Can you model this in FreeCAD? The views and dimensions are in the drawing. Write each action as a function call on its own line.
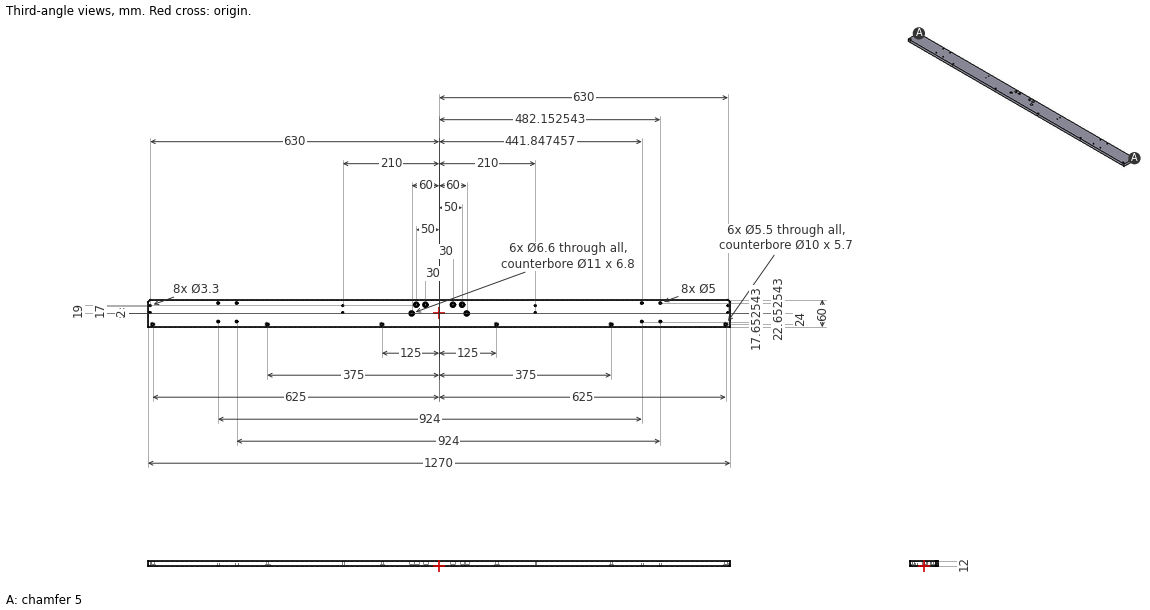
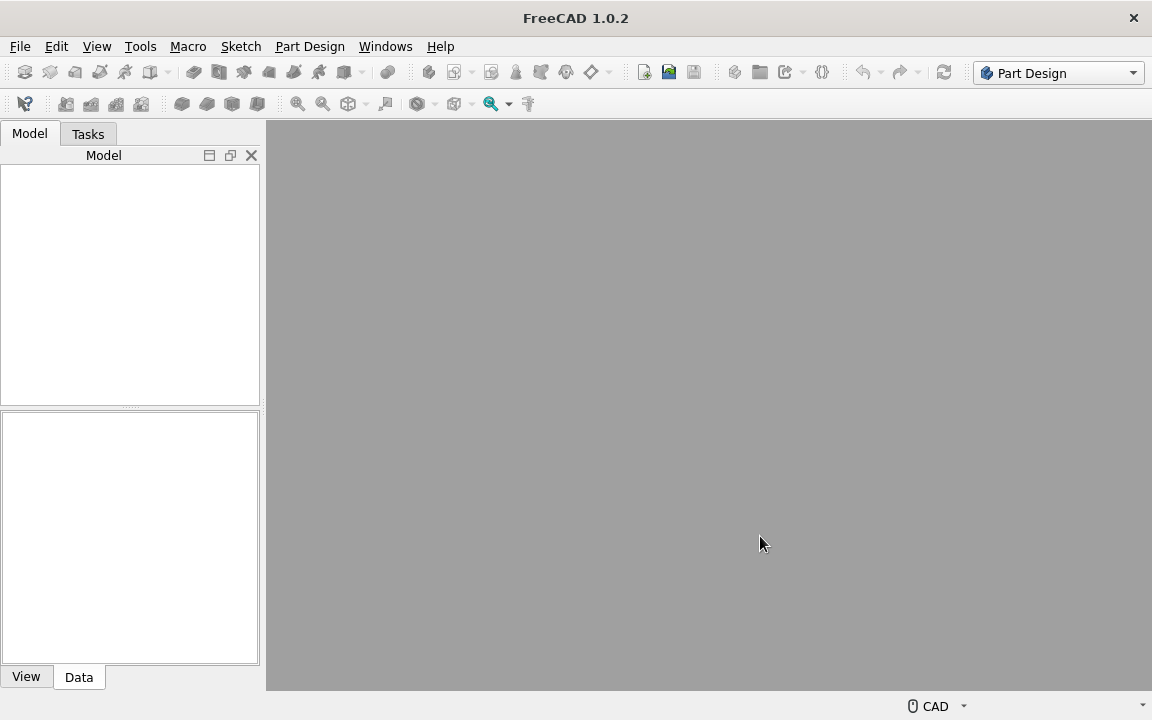
click(644, 72)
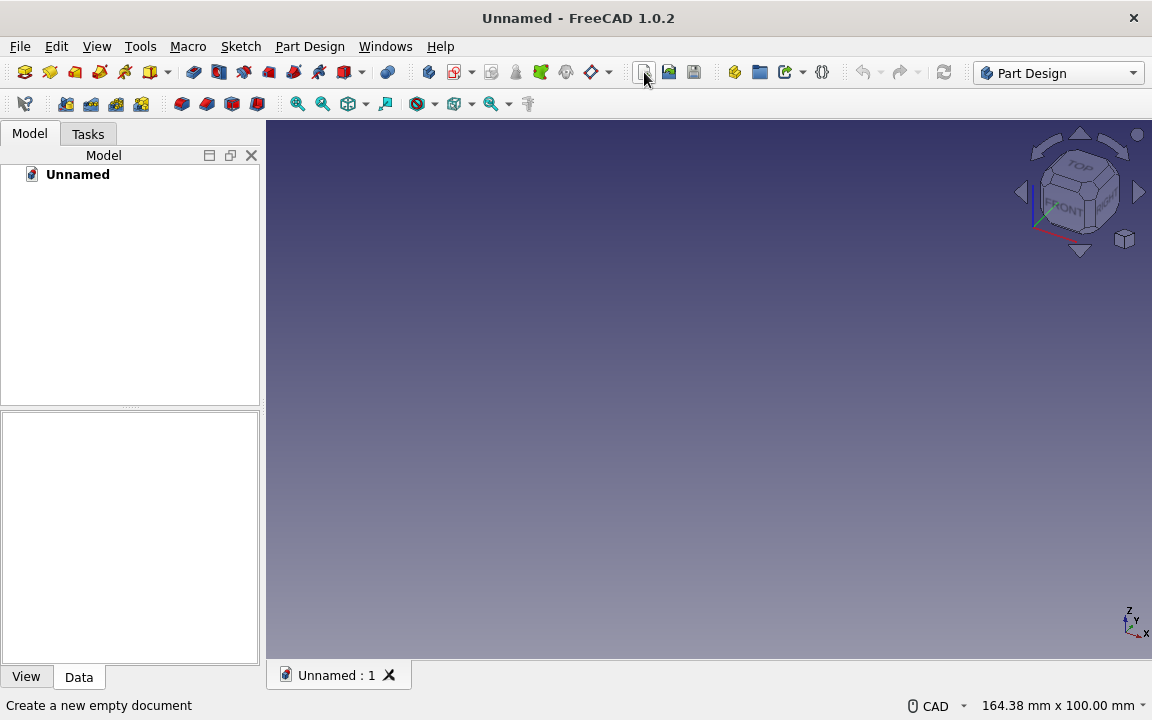
click(454, 72)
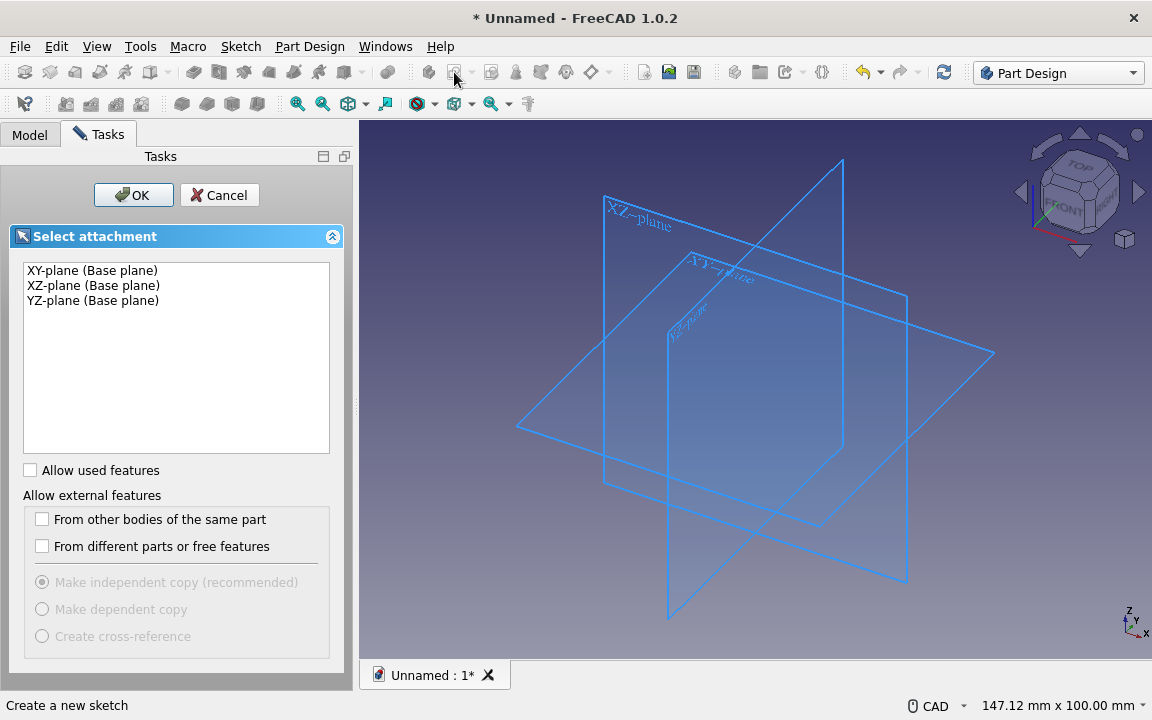
click(84, 270)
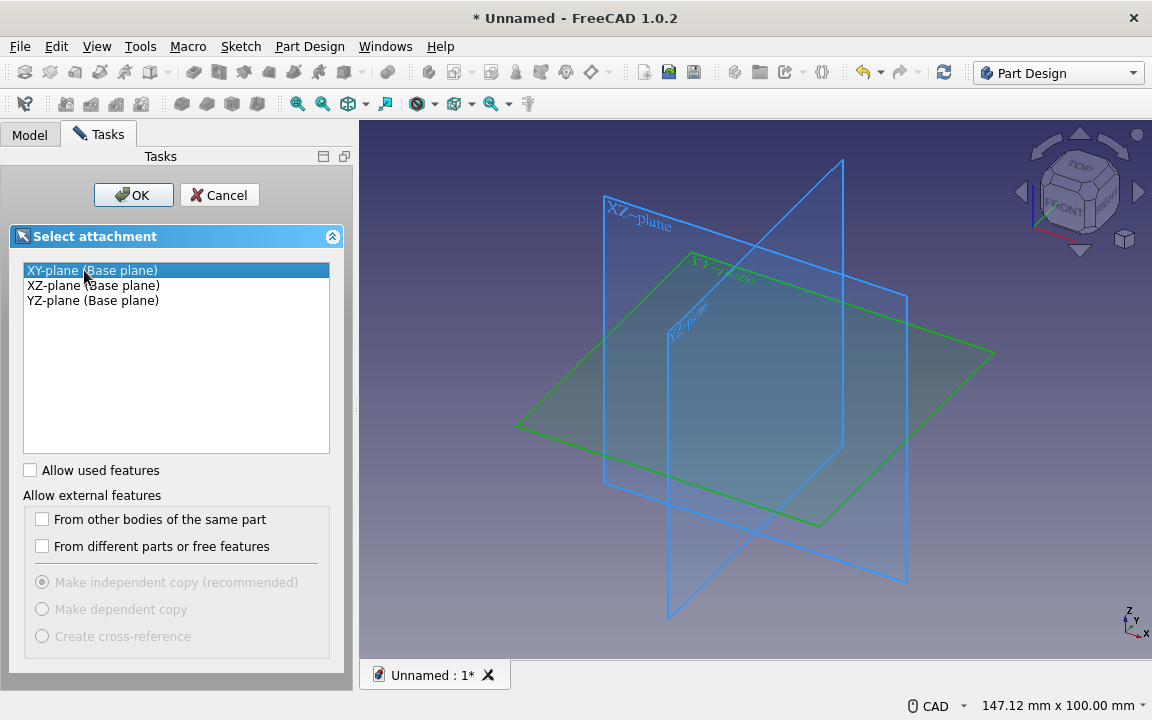
click(134, 195)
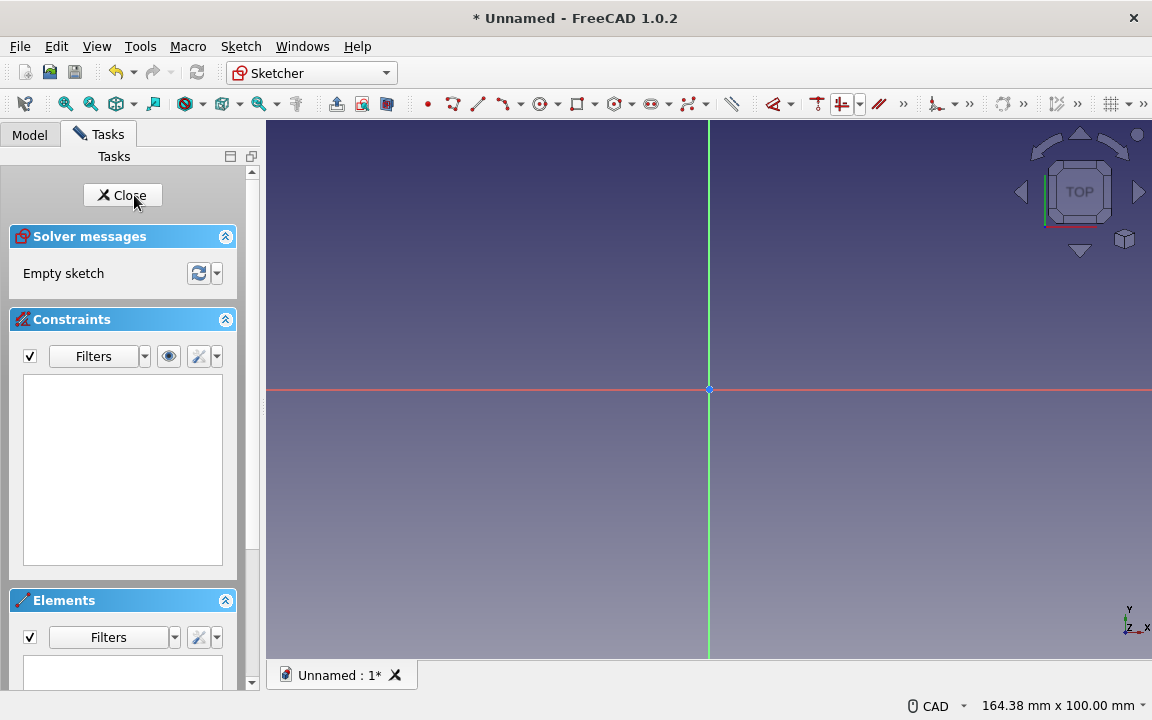
scroll(635, 390, down, 13)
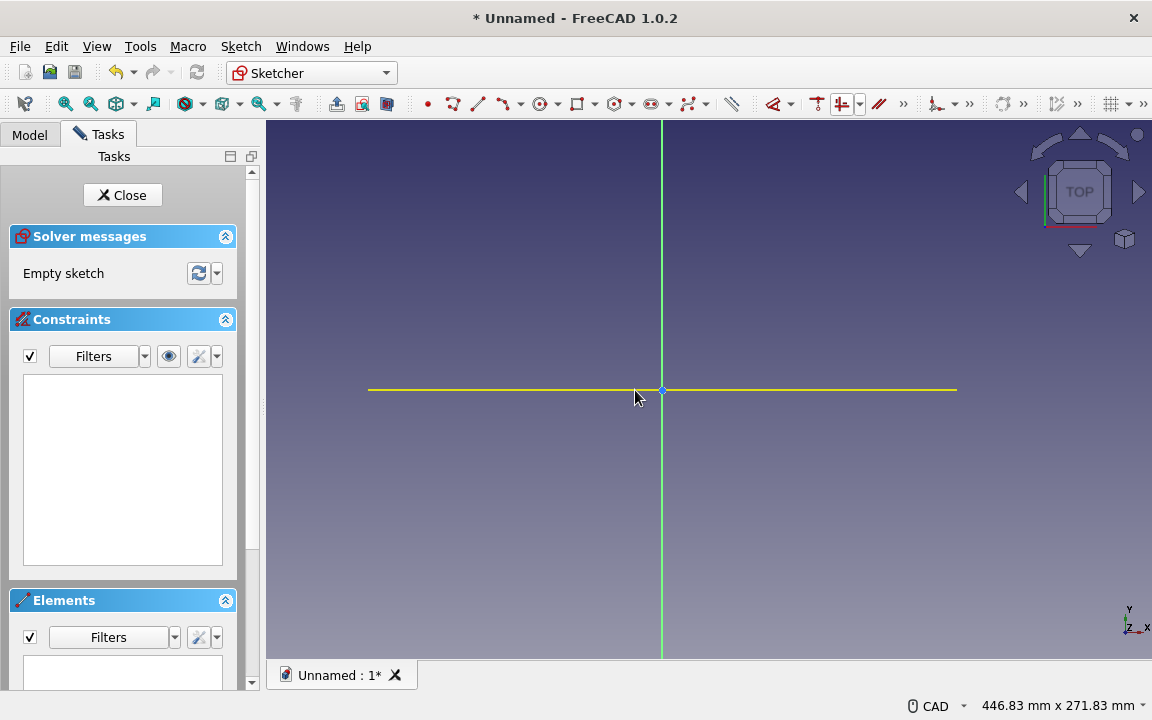
click(594, 104)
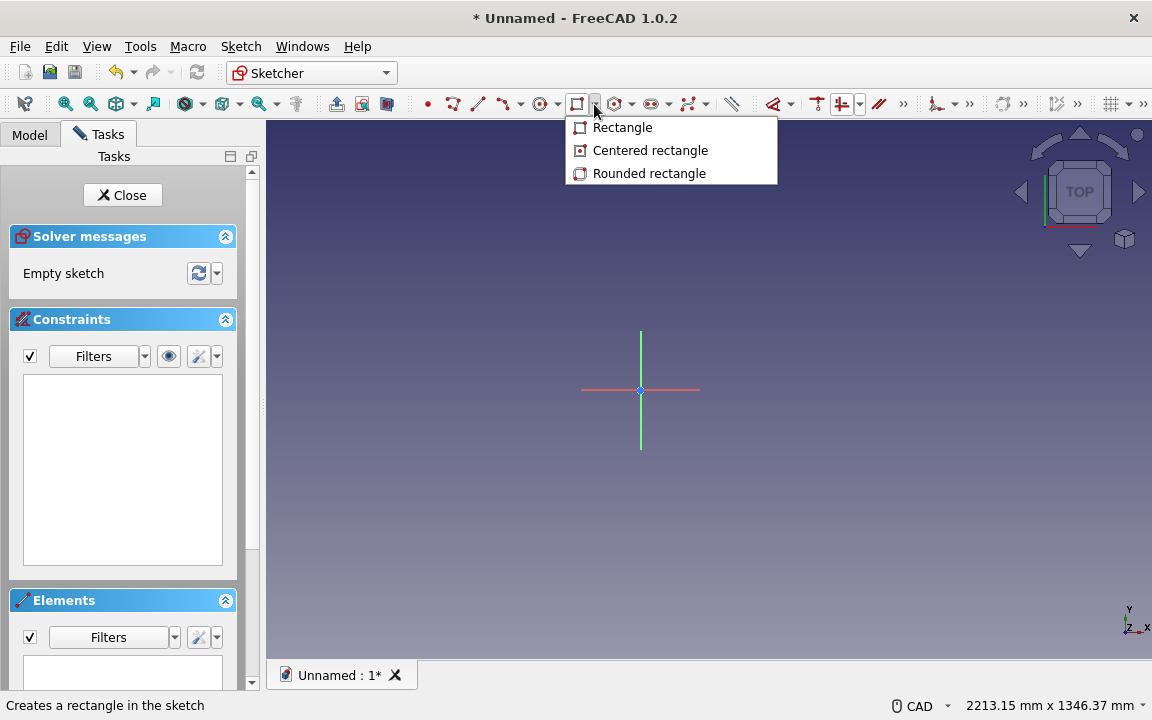
click(672, 150)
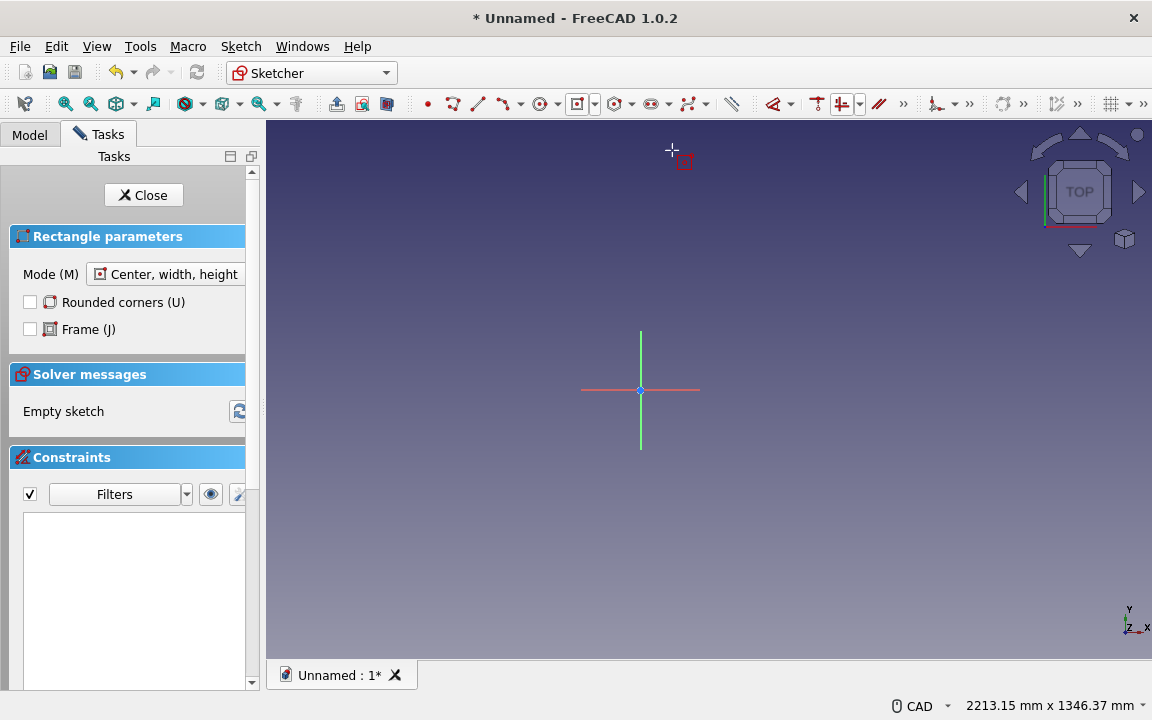
scroll(641, 390, up, 2)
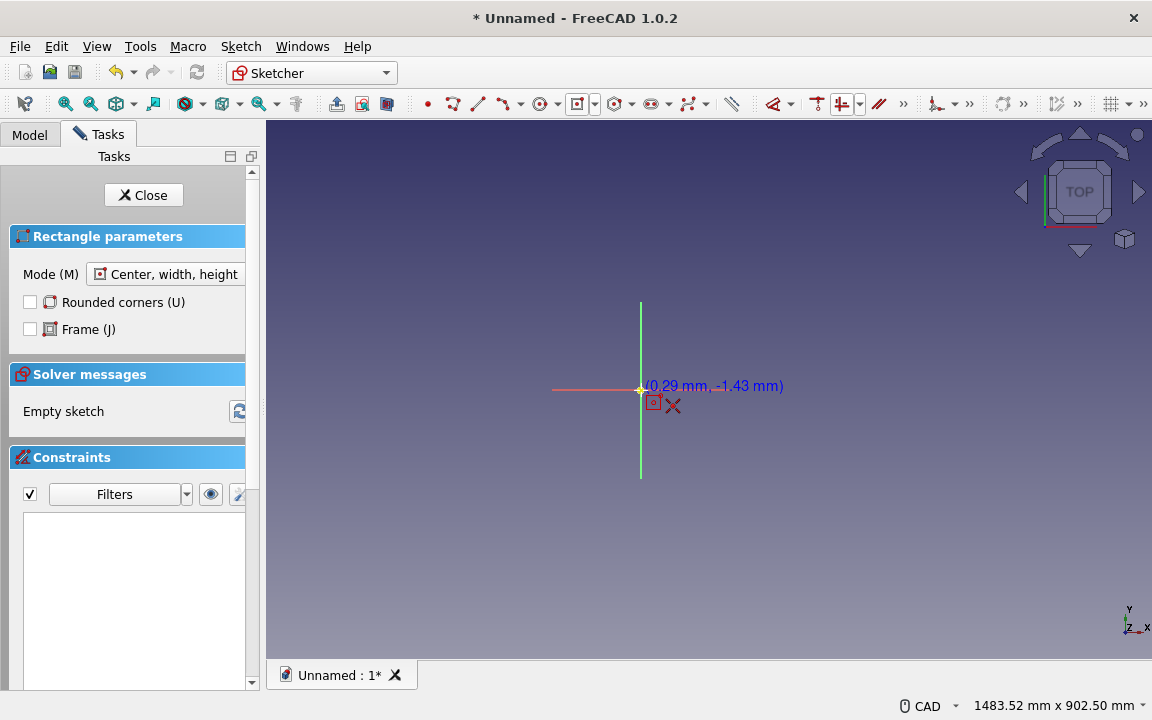
click(641, 390)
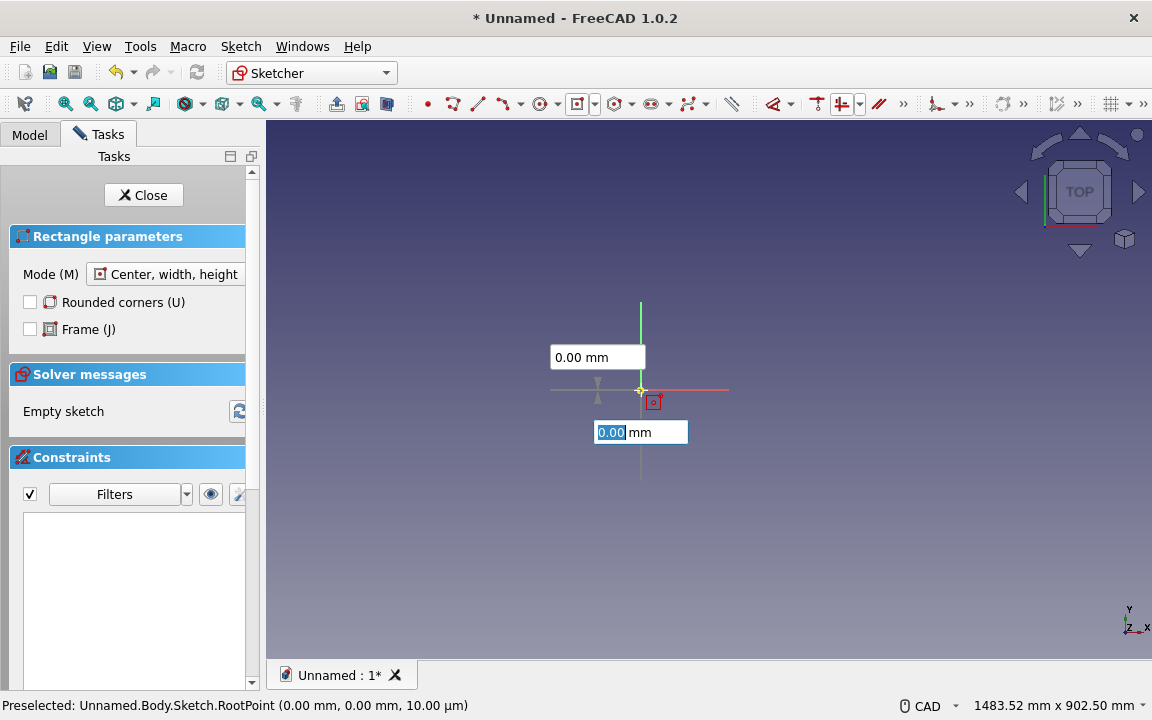
scroll(640, 388, down, 2)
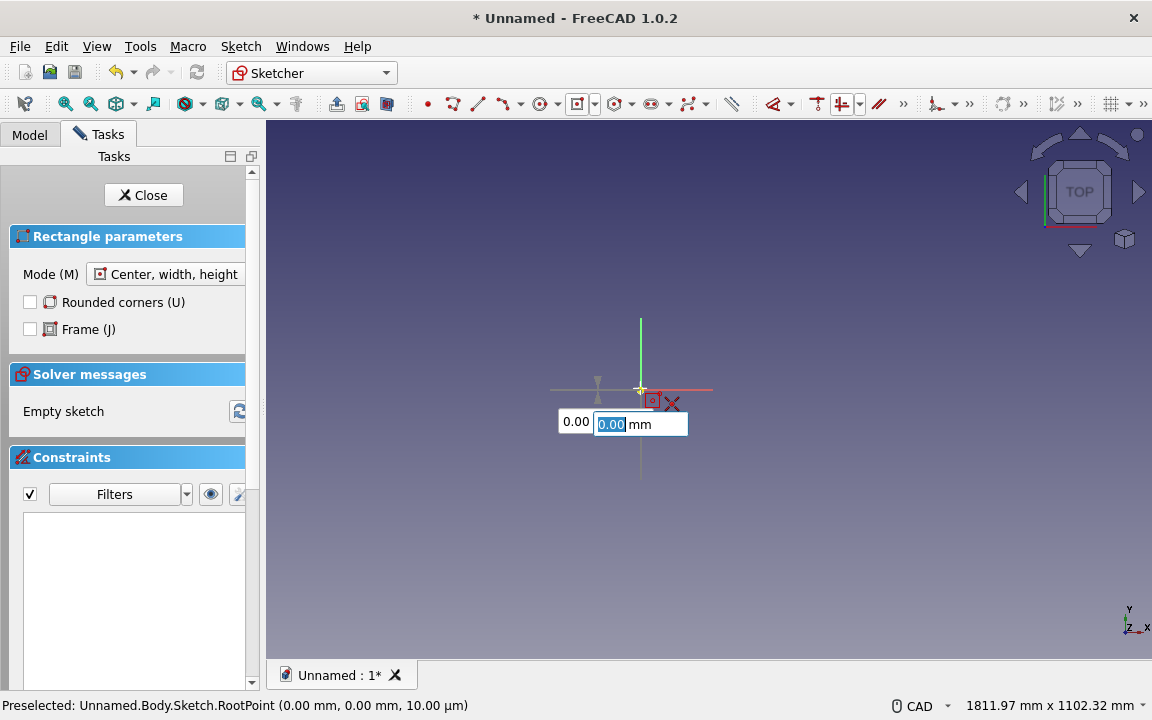
scroll(895, 378, up, 2)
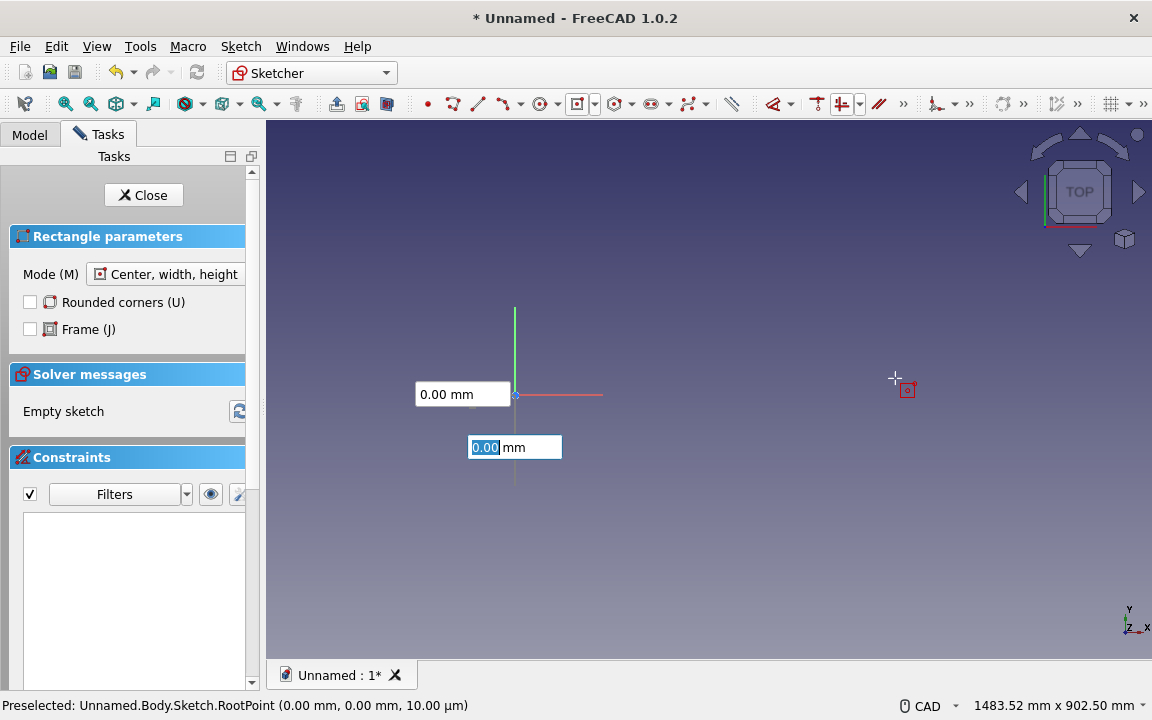
click(894, 377)
key(Escape)